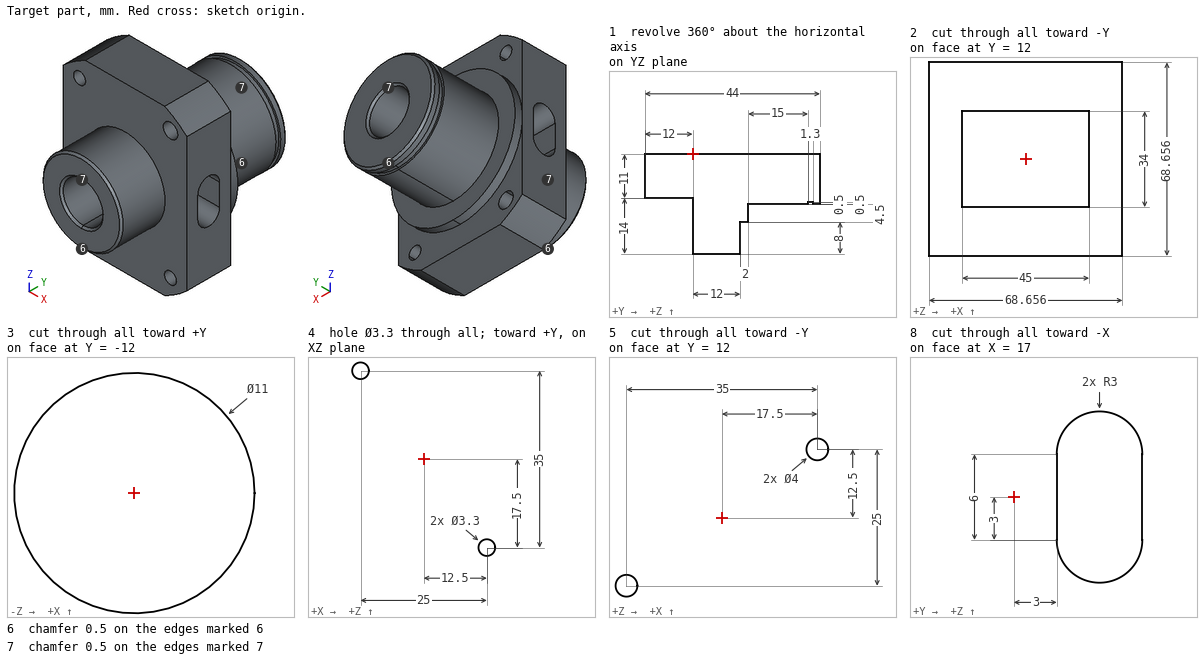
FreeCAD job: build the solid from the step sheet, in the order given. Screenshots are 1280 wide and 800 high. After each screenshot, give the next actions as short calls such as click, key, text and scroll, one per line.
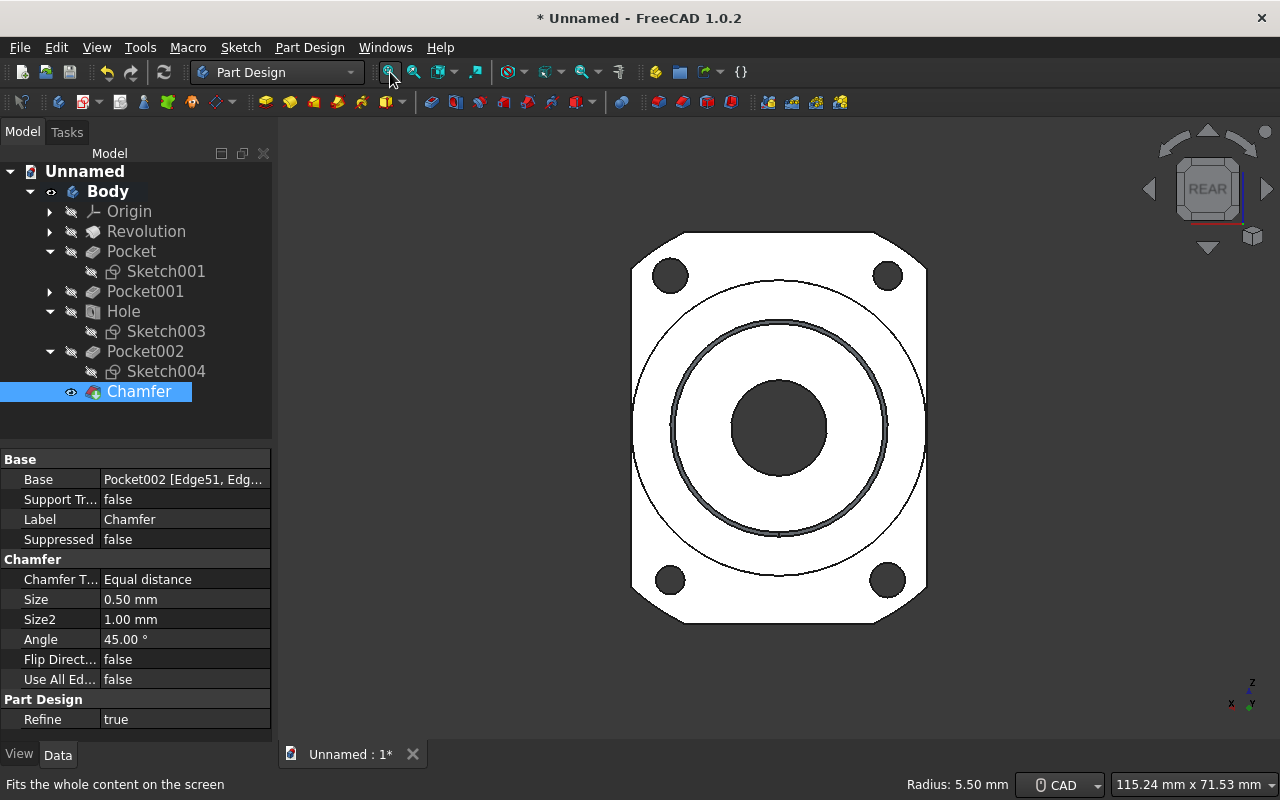
click(779, 379, ctrl)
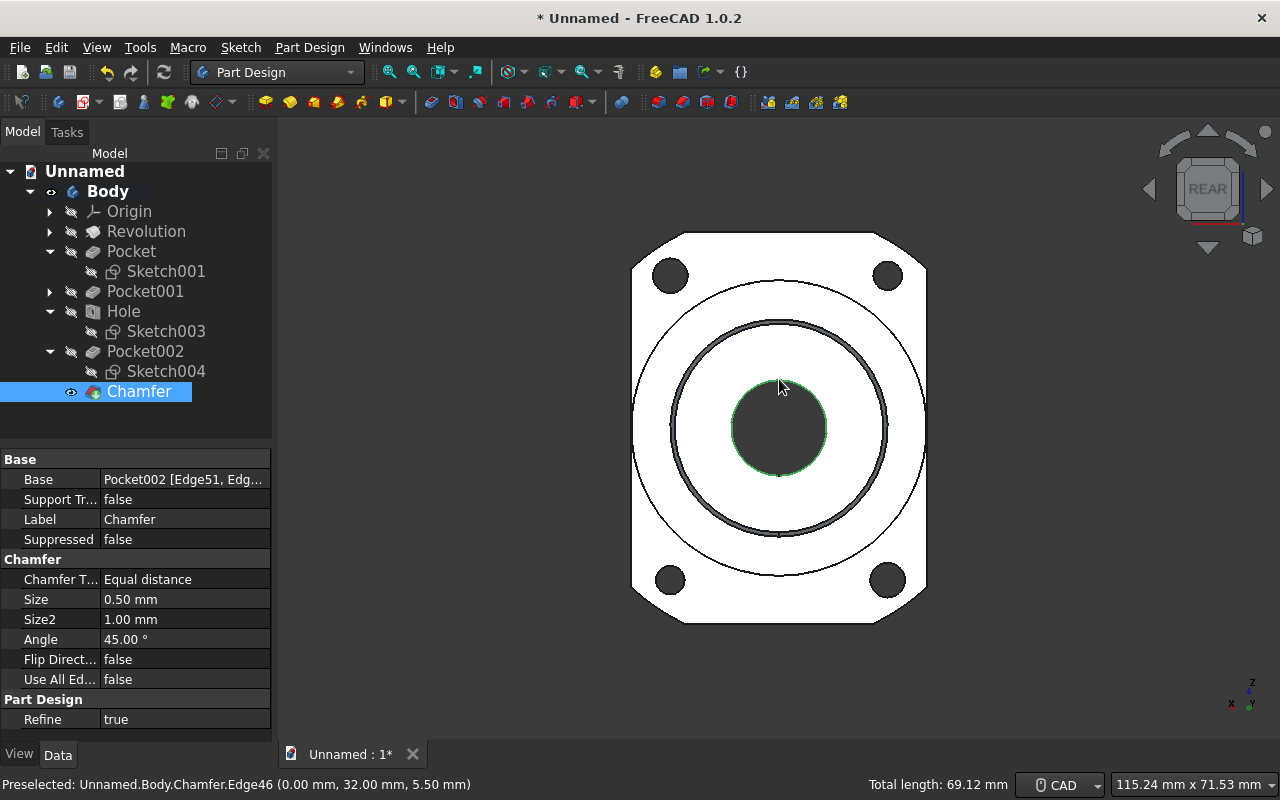
click(684, 102)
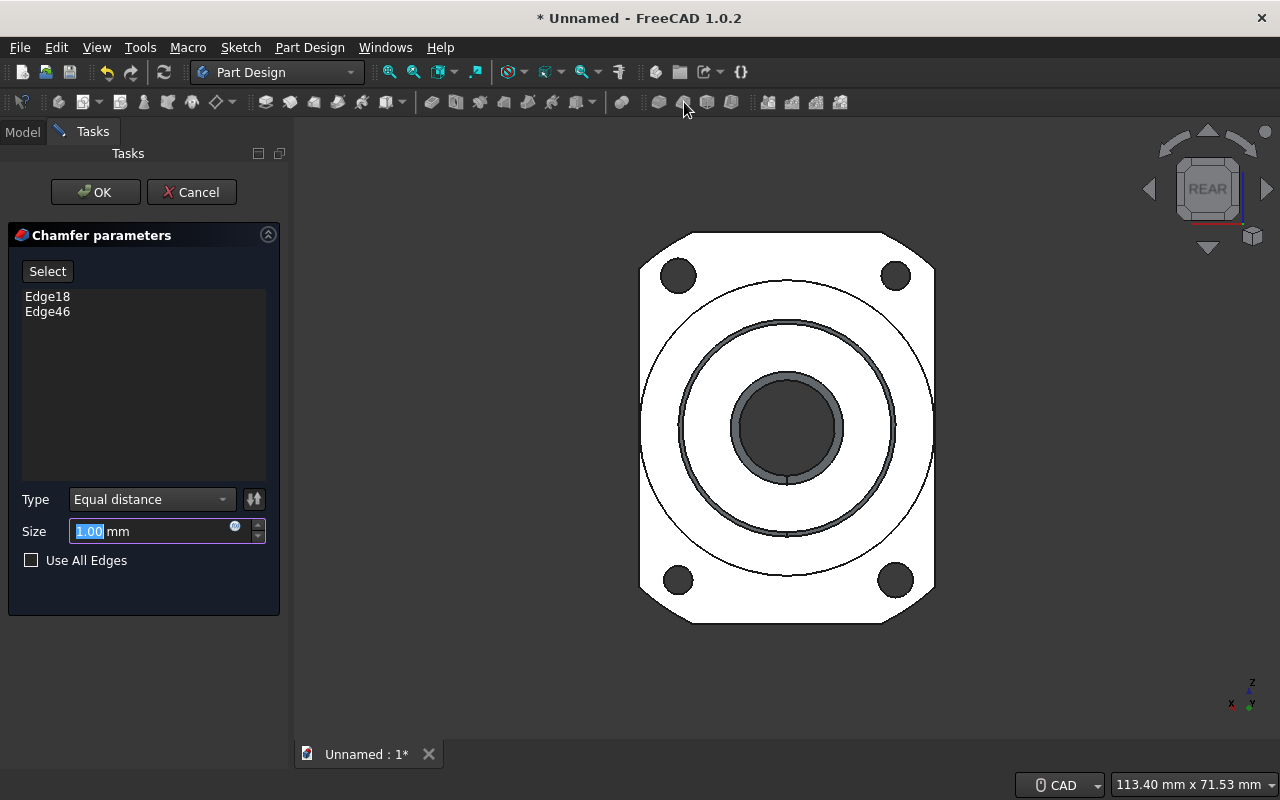
text(0.5)
key(Tab)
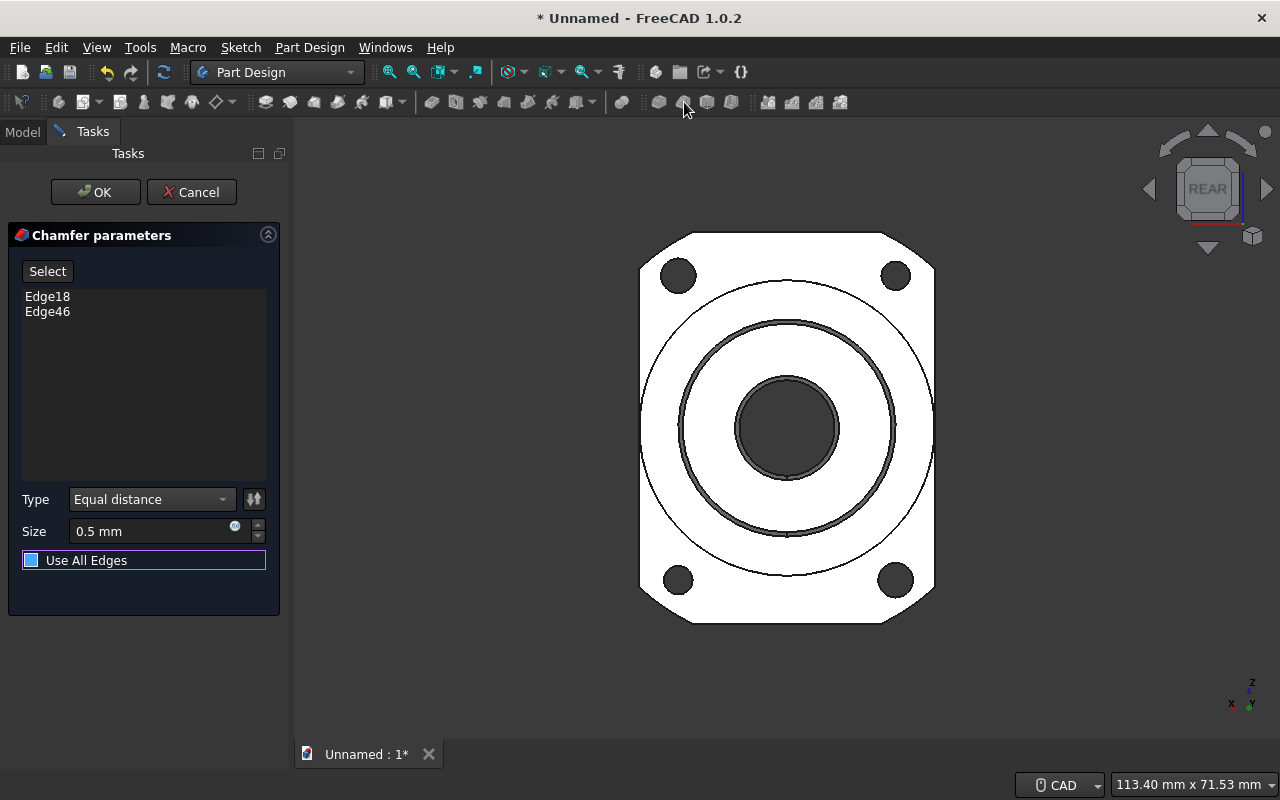
click(96, 192)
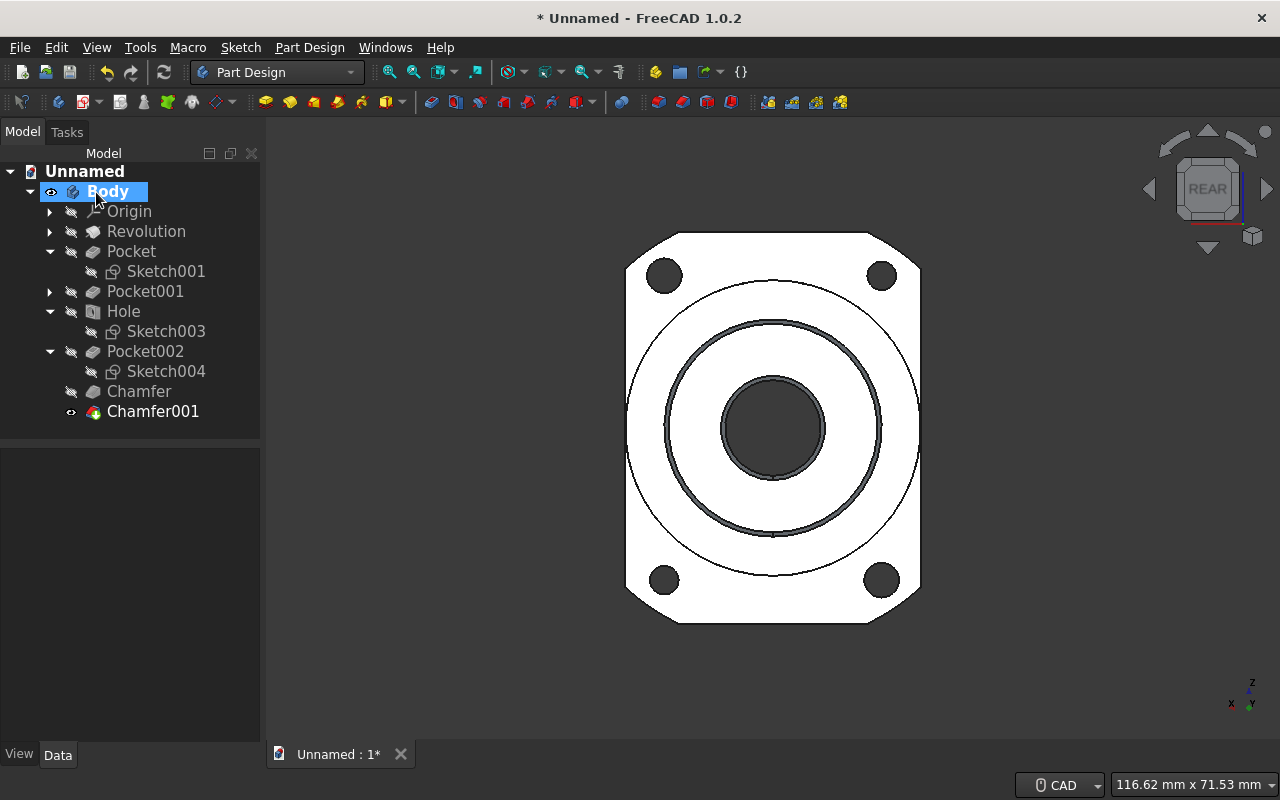
key(0)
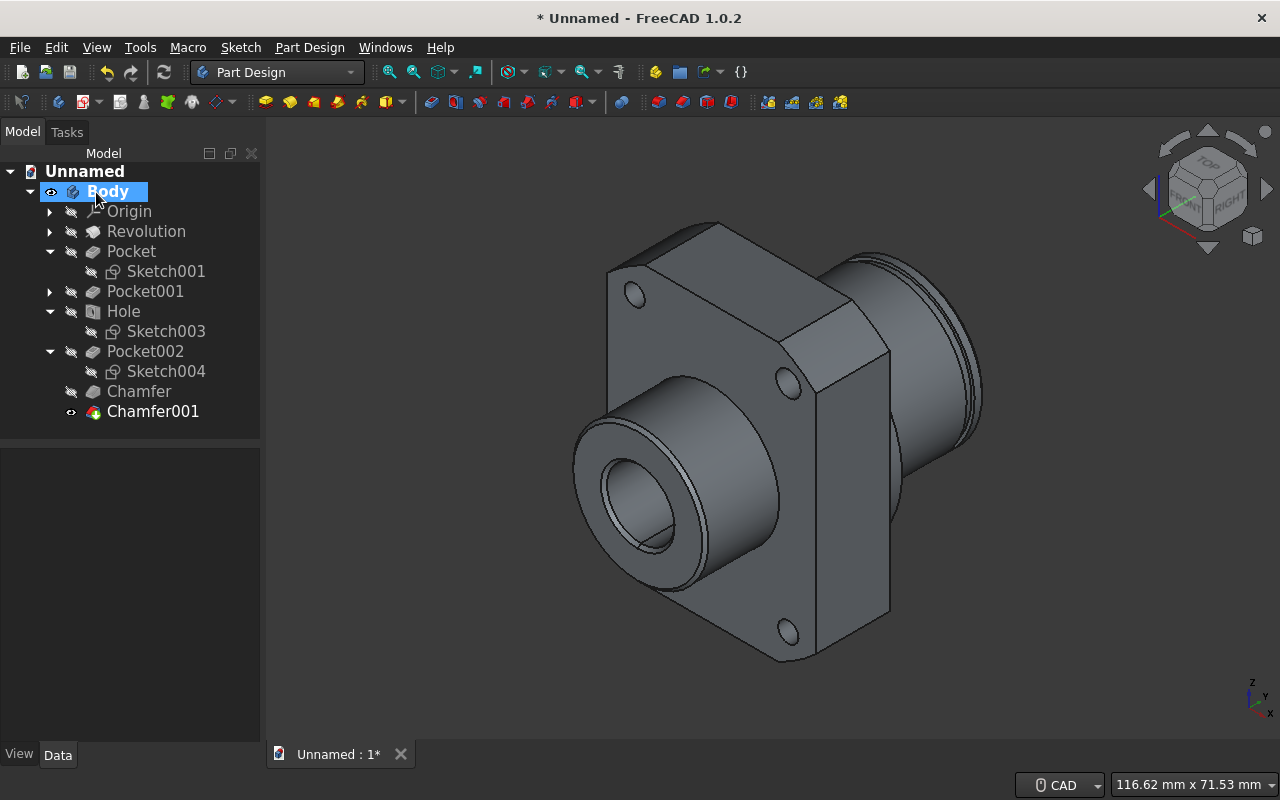
click(853, 576)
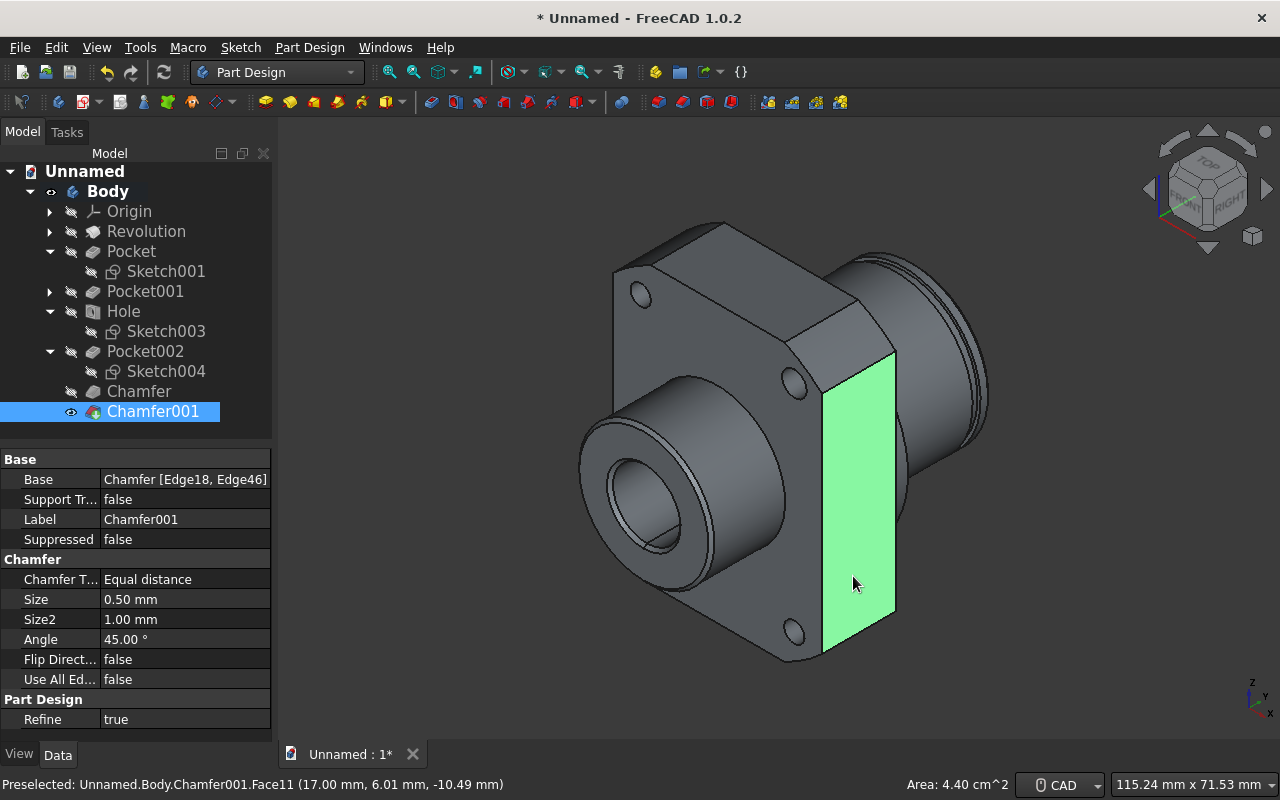
click(84, 102)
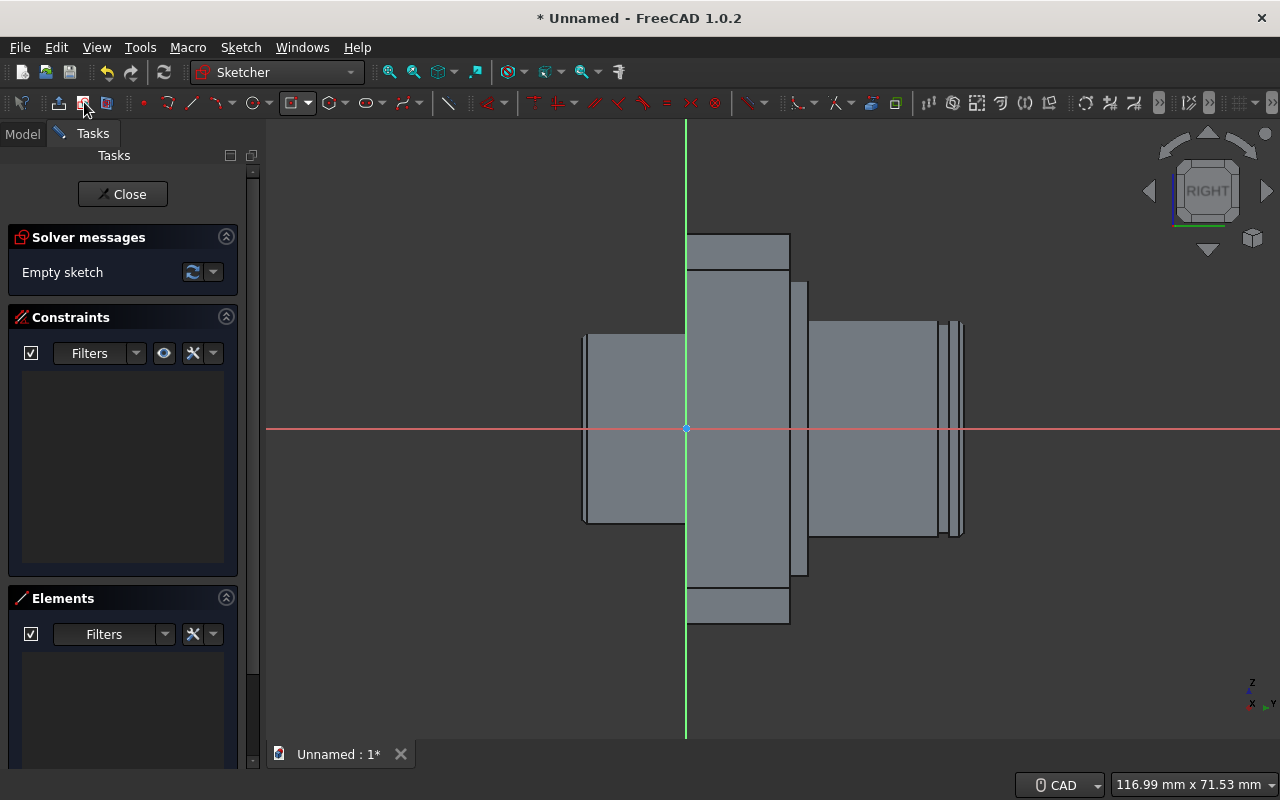
scroll(732, 429, up, 7)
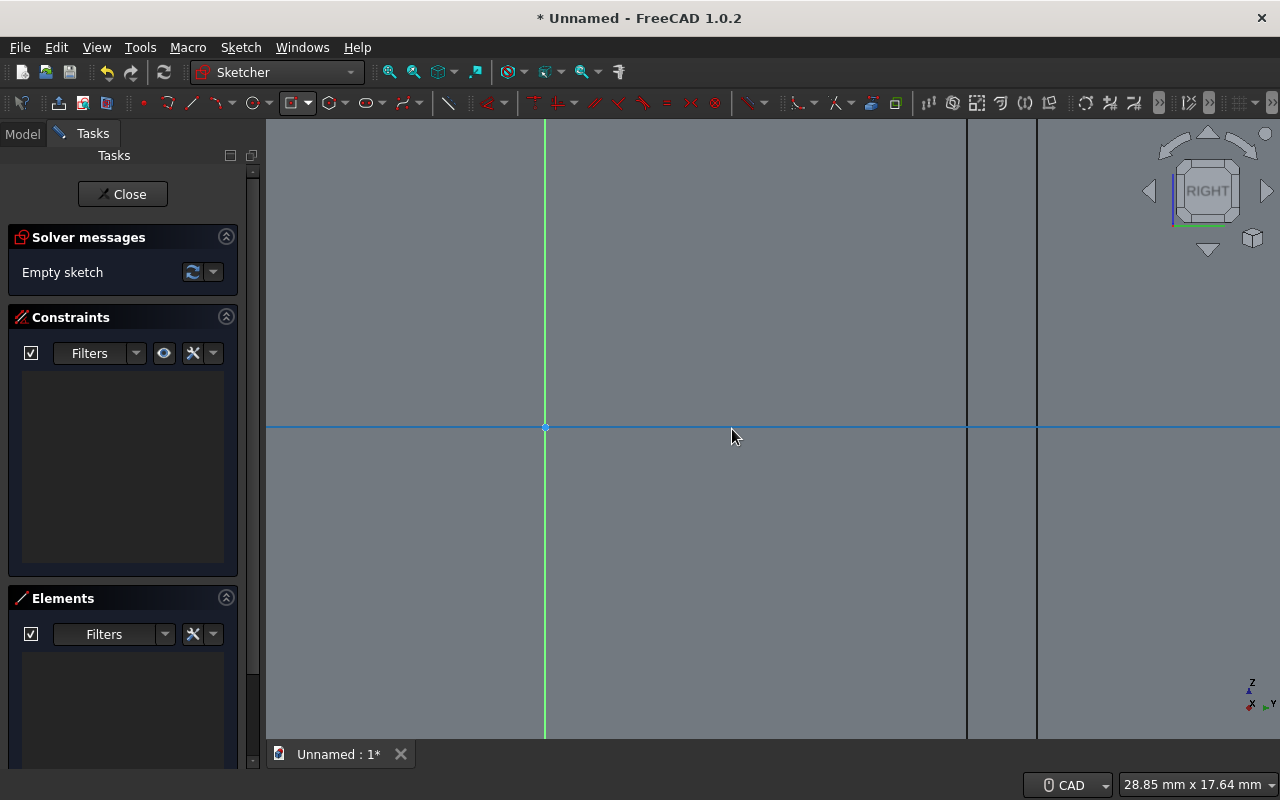
click(366, 104)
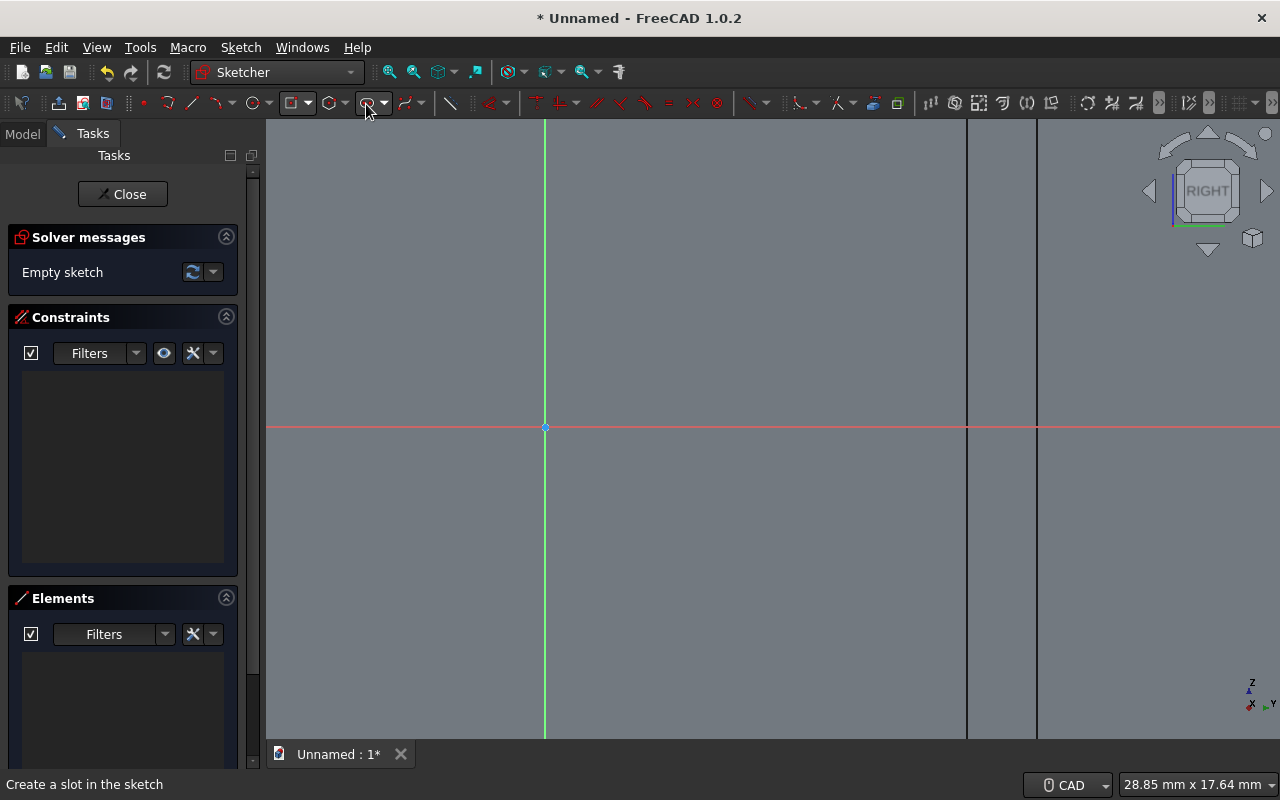
click(756, 533)